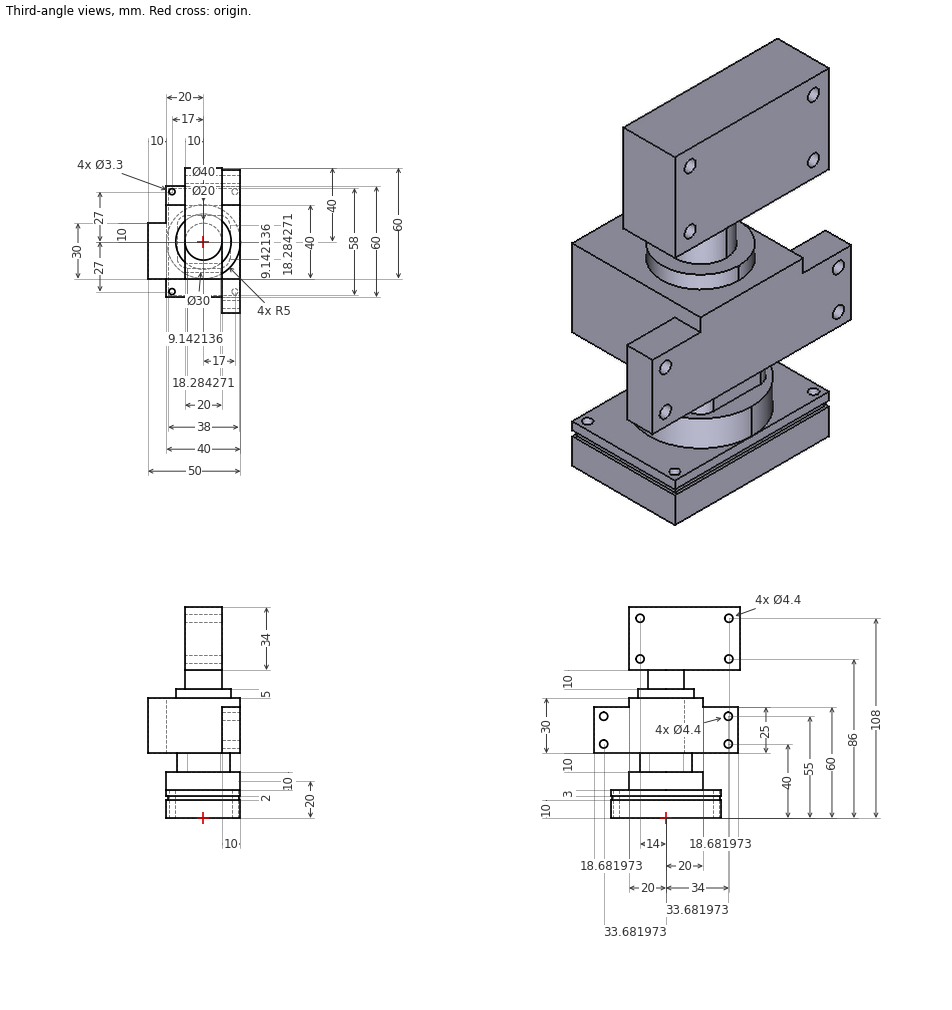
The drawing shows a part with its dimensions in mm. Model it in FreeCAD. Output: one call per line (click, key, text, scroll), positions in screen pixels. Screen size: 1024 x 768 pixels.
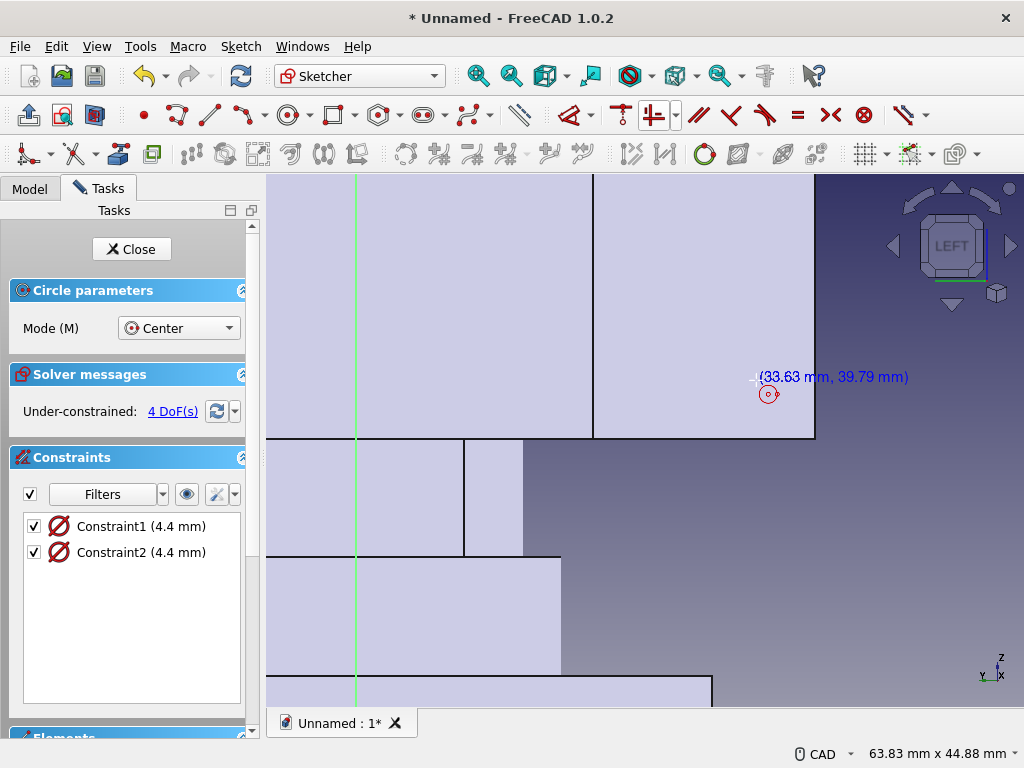
click(756, 379)
move(774, 361)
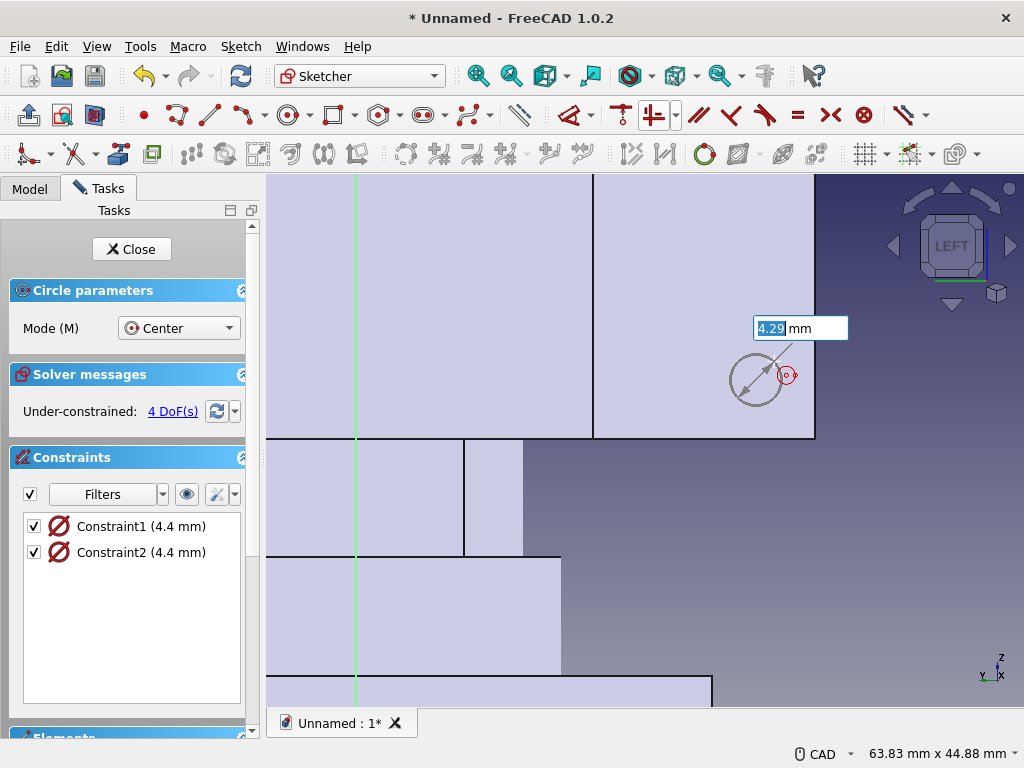
text(4.4)
key(Return)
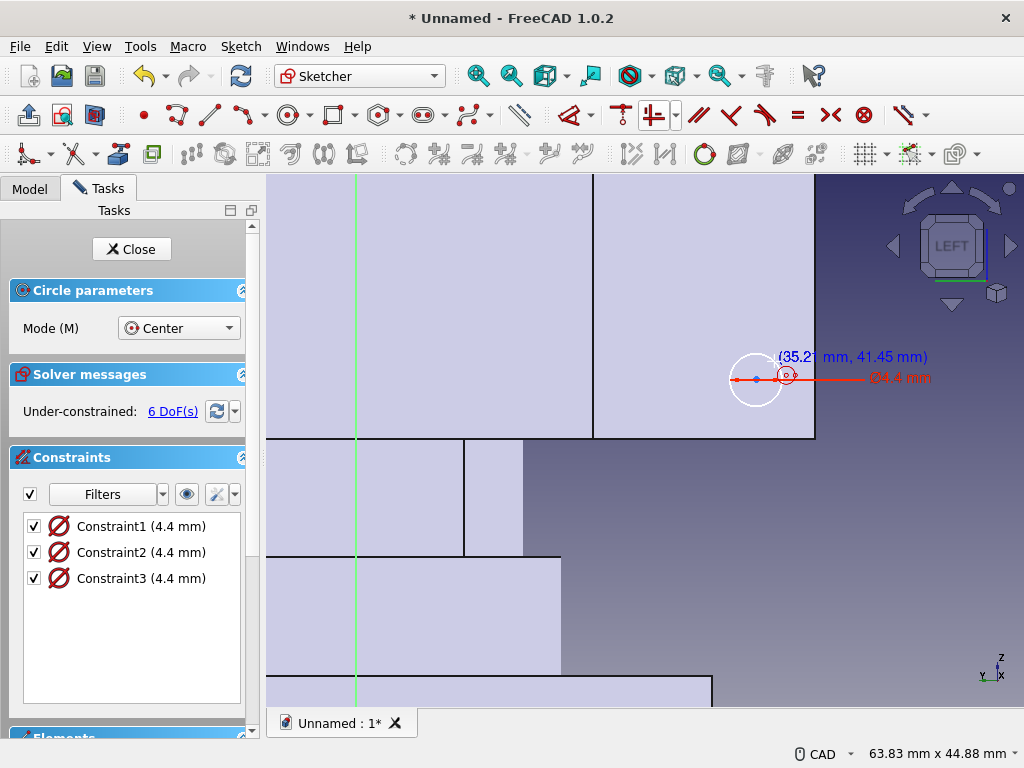
scroll(757, 380, down, 4)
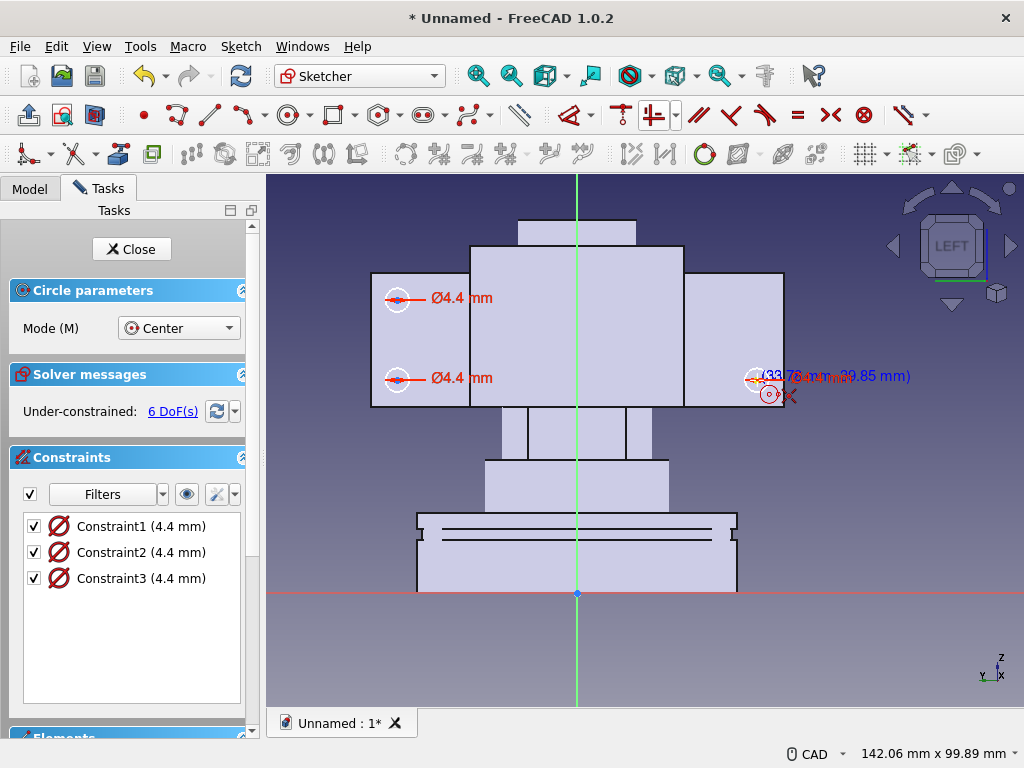
scroll(757, 300, up, 4)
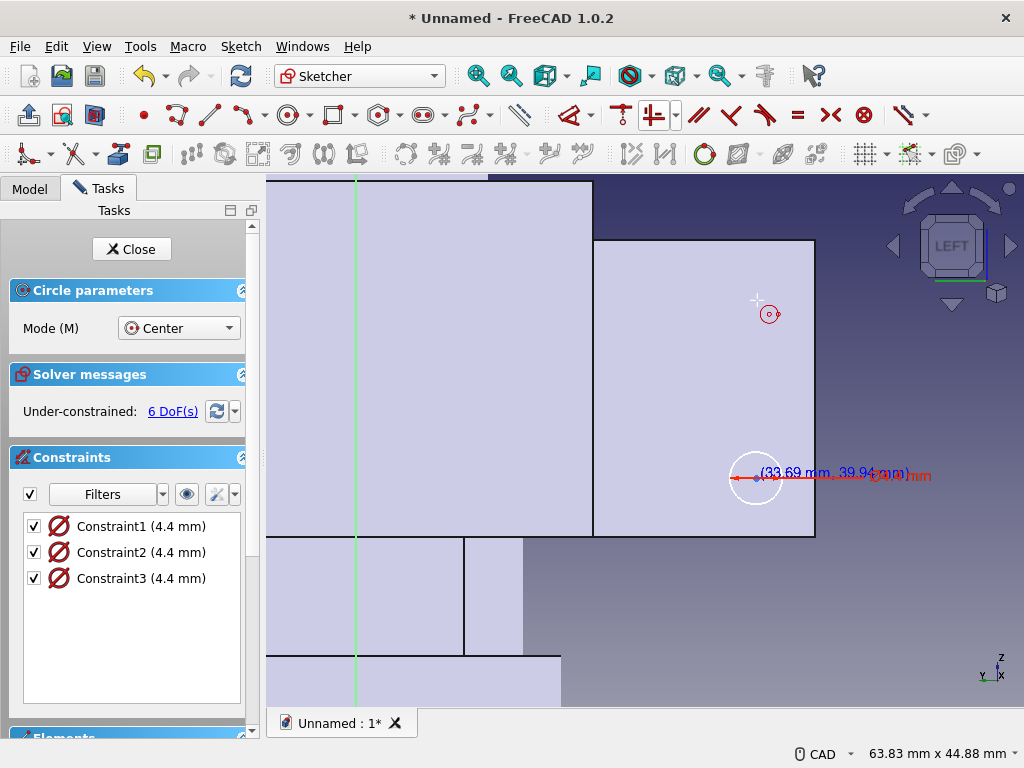
click(756, 299)
move(774, 281)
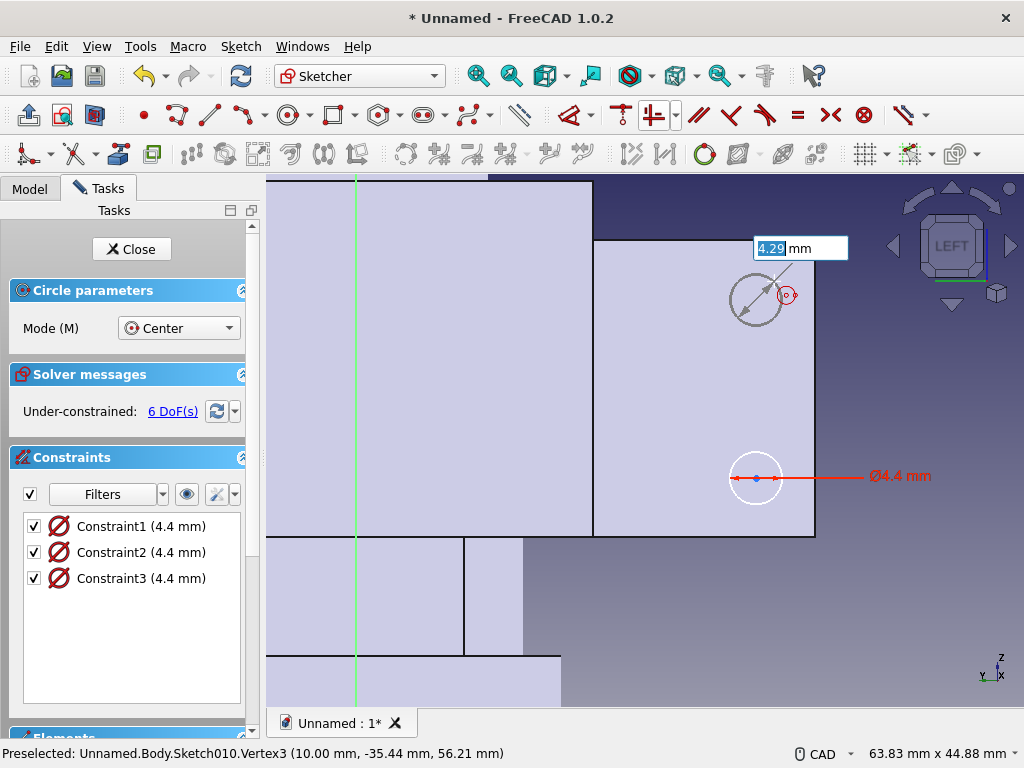
text(4.4)
key(Return)
key(Escape)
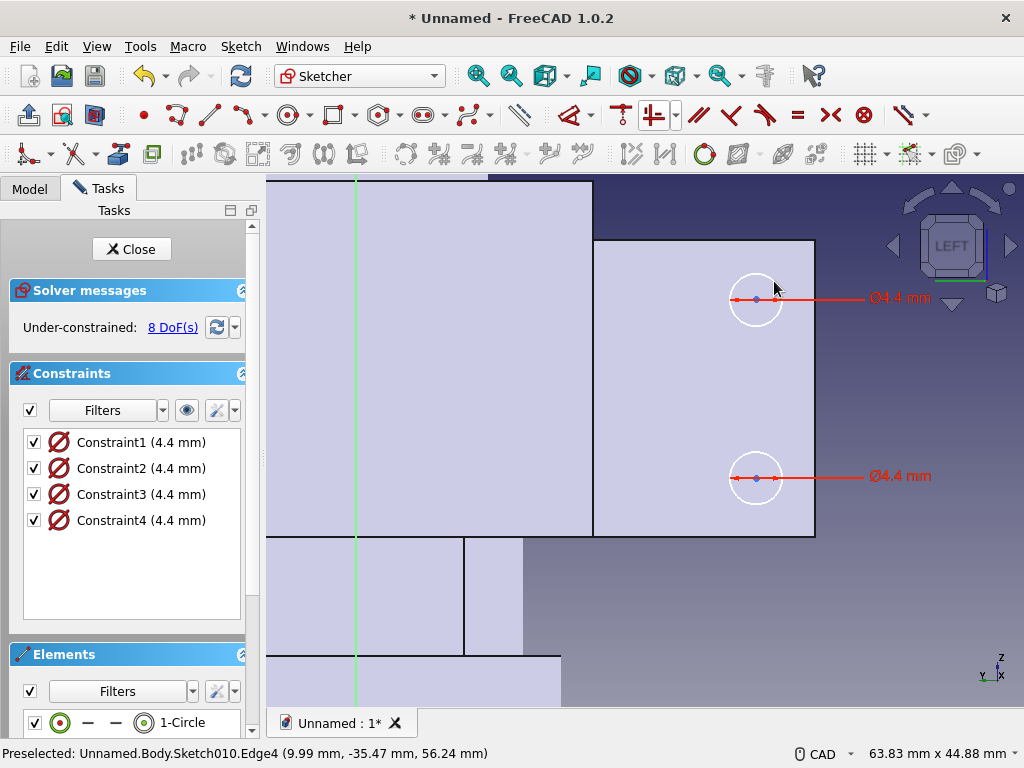
scroll(757, 300, down, 4)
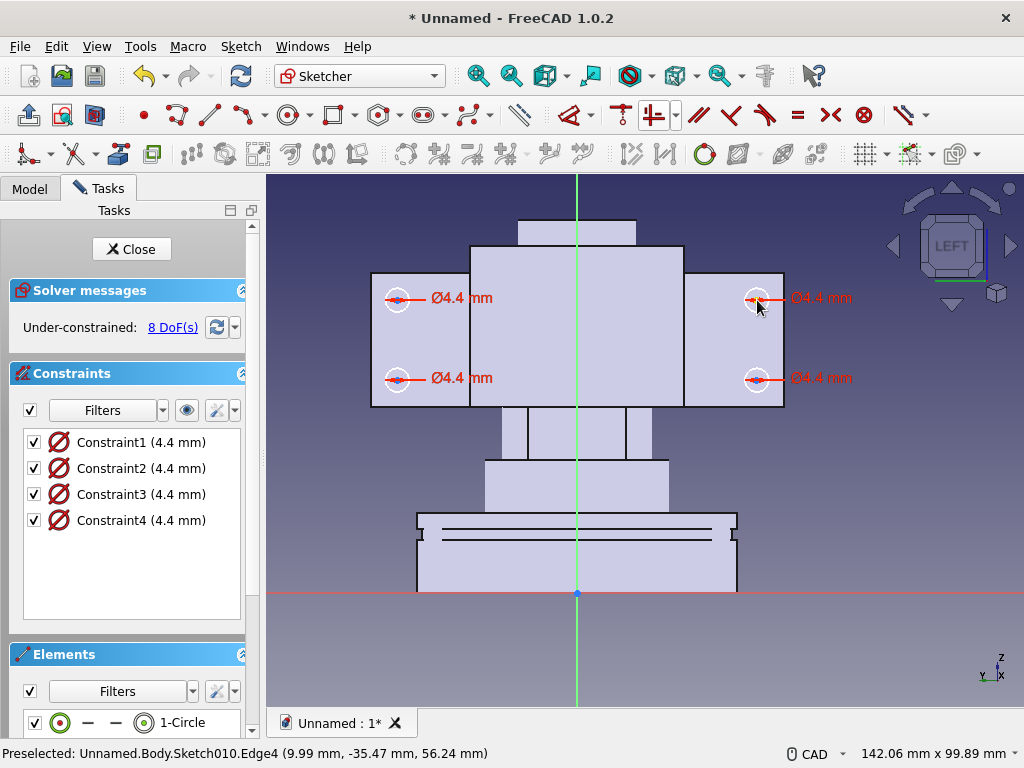
click(397, 300)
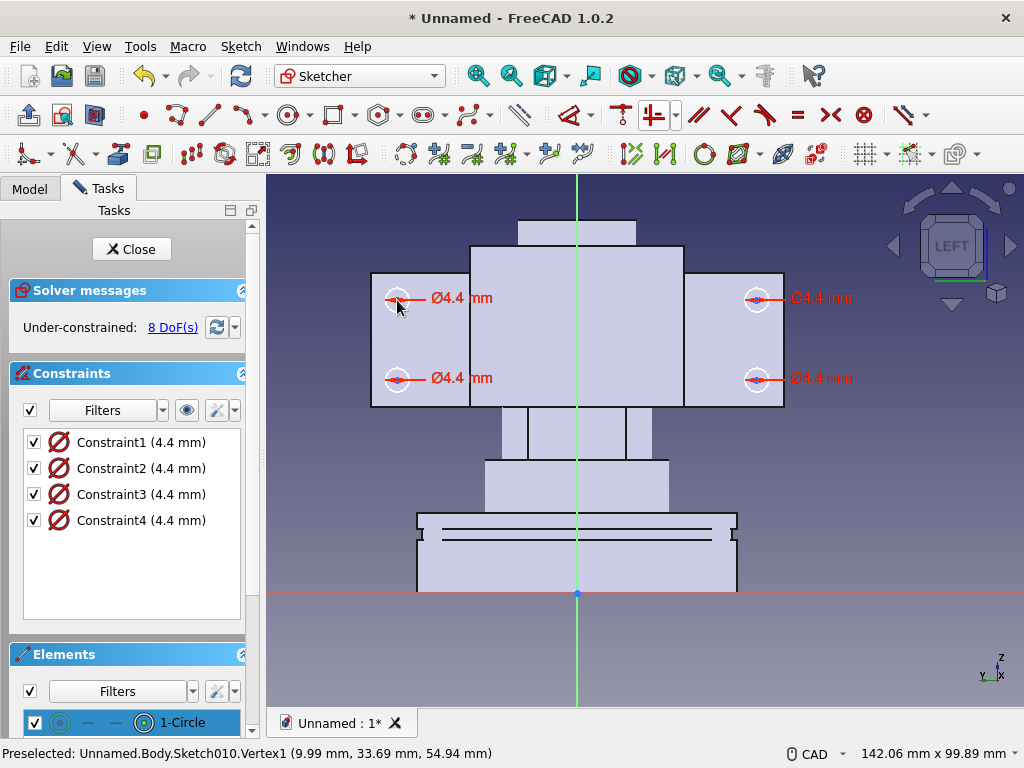
click(397, 380)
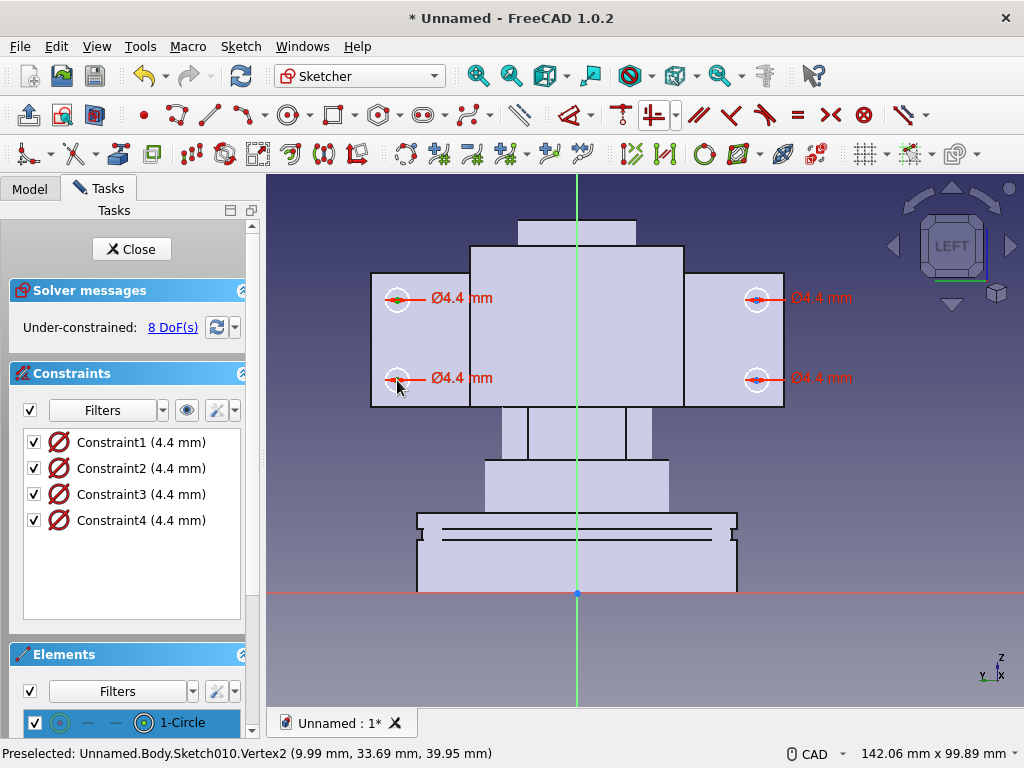
key(v)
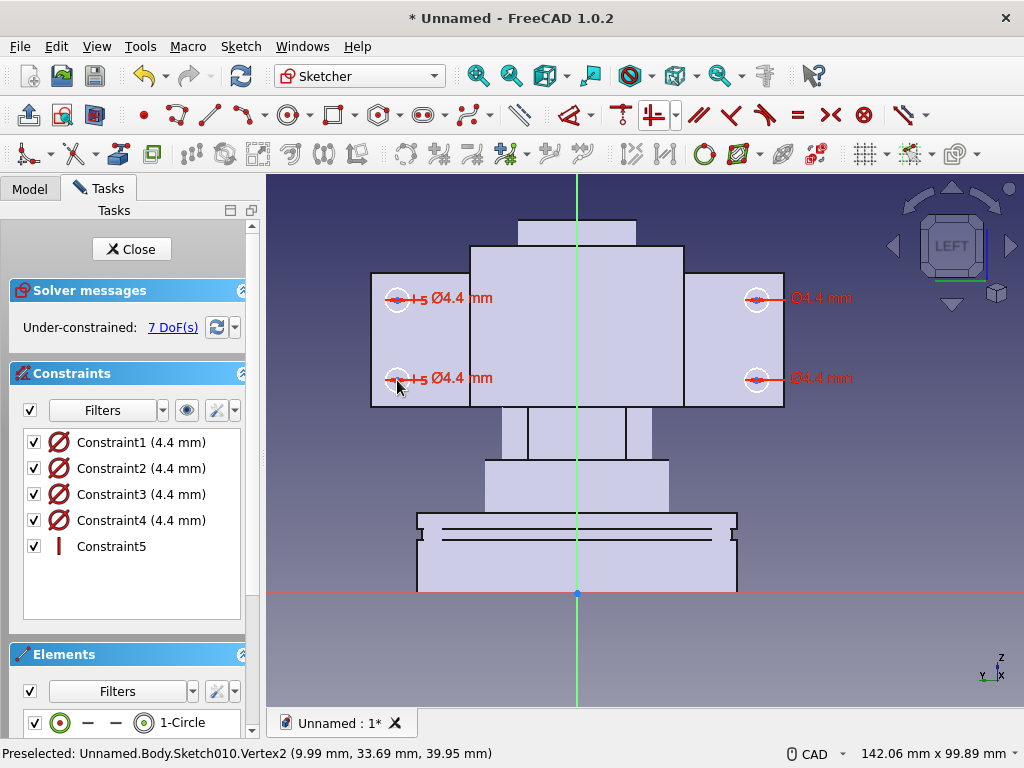
click(397, 380)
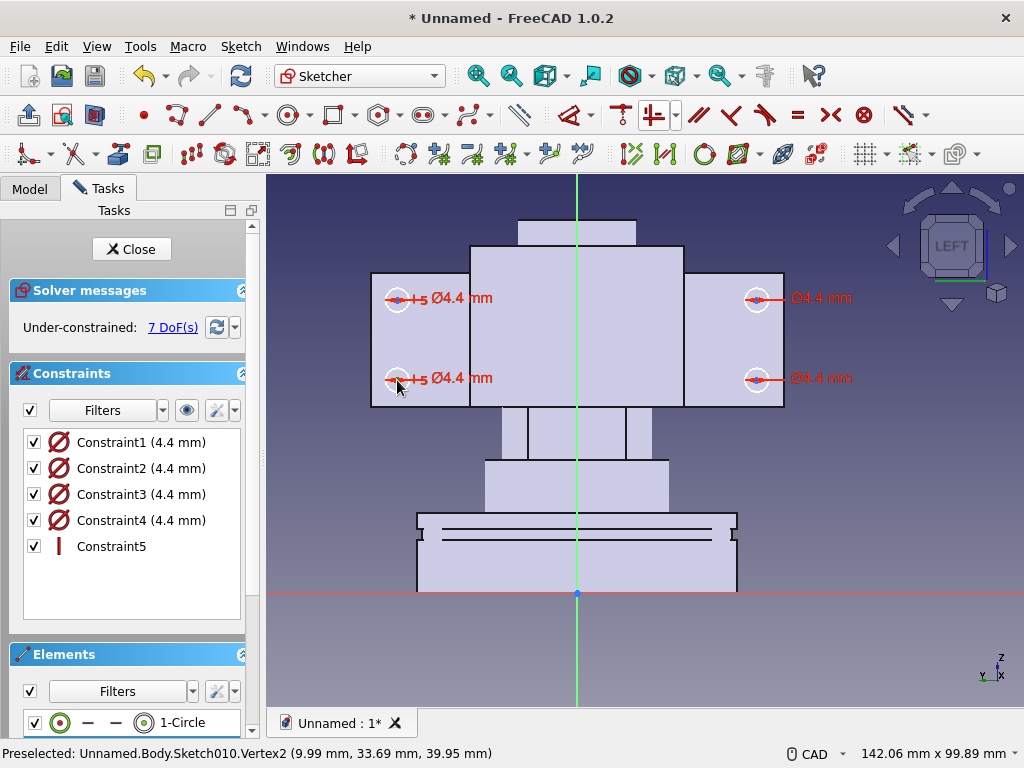
click(757, 380)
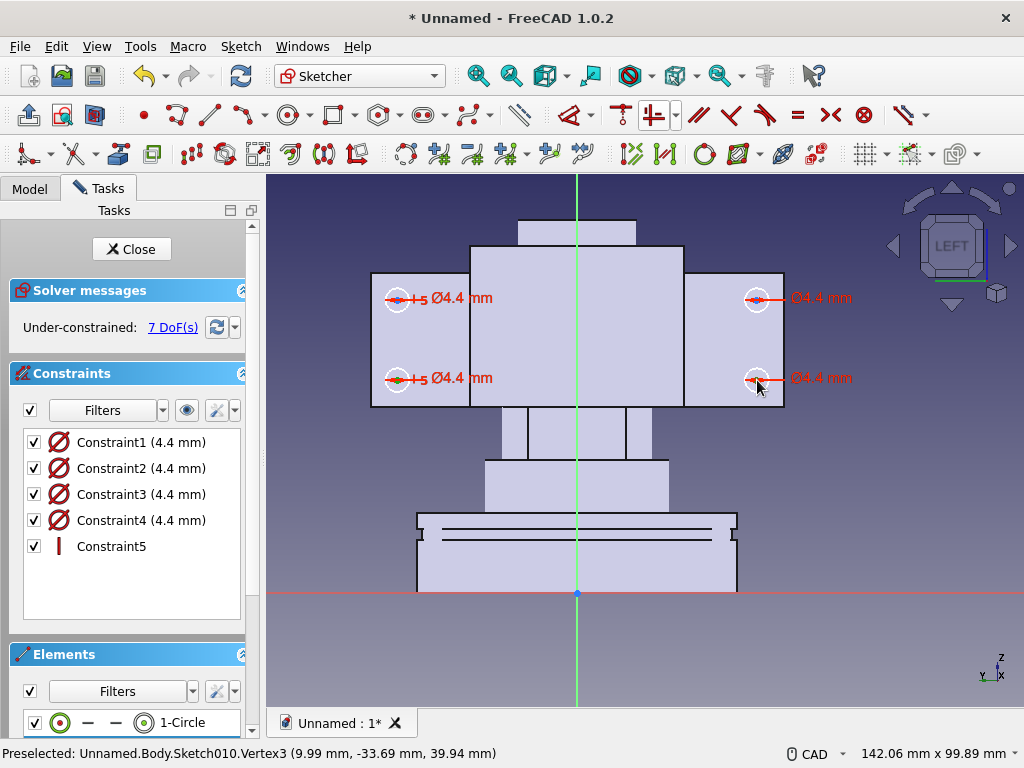
click(676, 116)